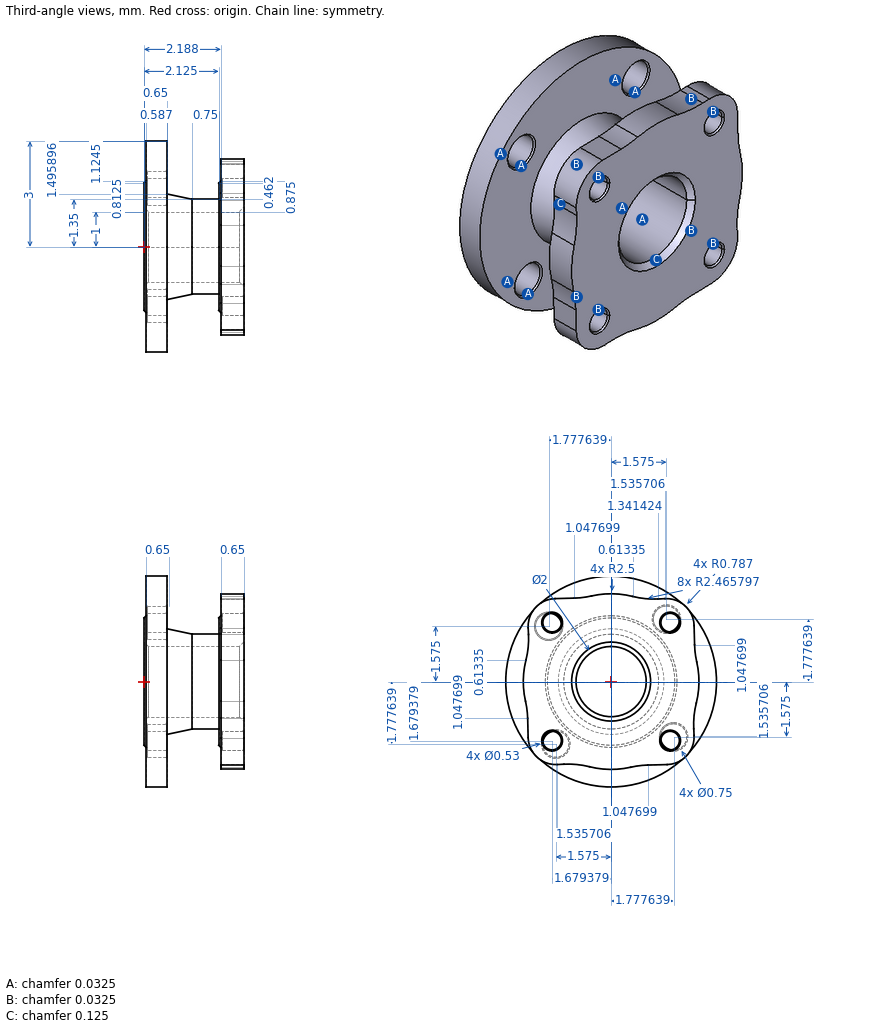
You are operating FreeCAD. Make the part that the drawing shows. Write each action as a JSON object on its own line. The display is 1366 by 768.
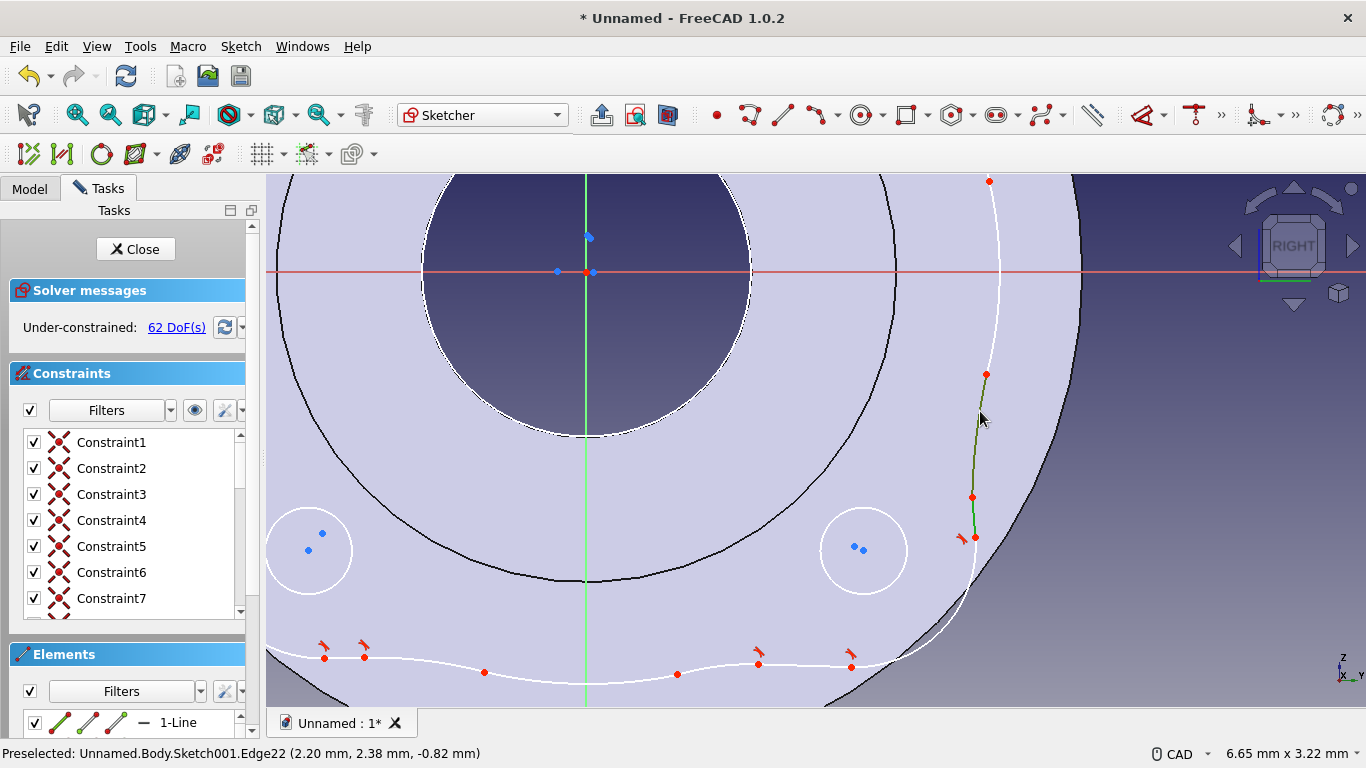
{"action": "key", "text": "t"}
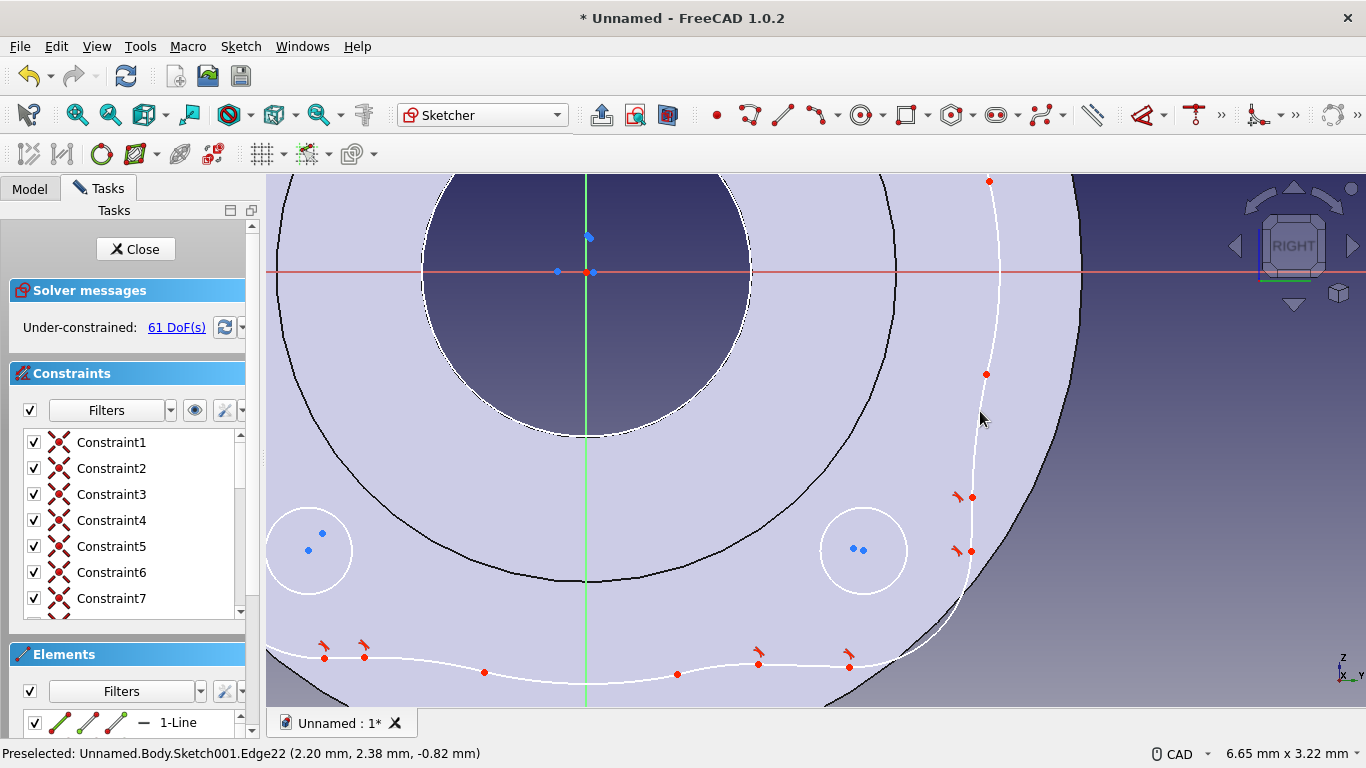
{"action": "scroll", "coordinate": [879, 578], "scroll_direction": "down", "scroll_amount": 4}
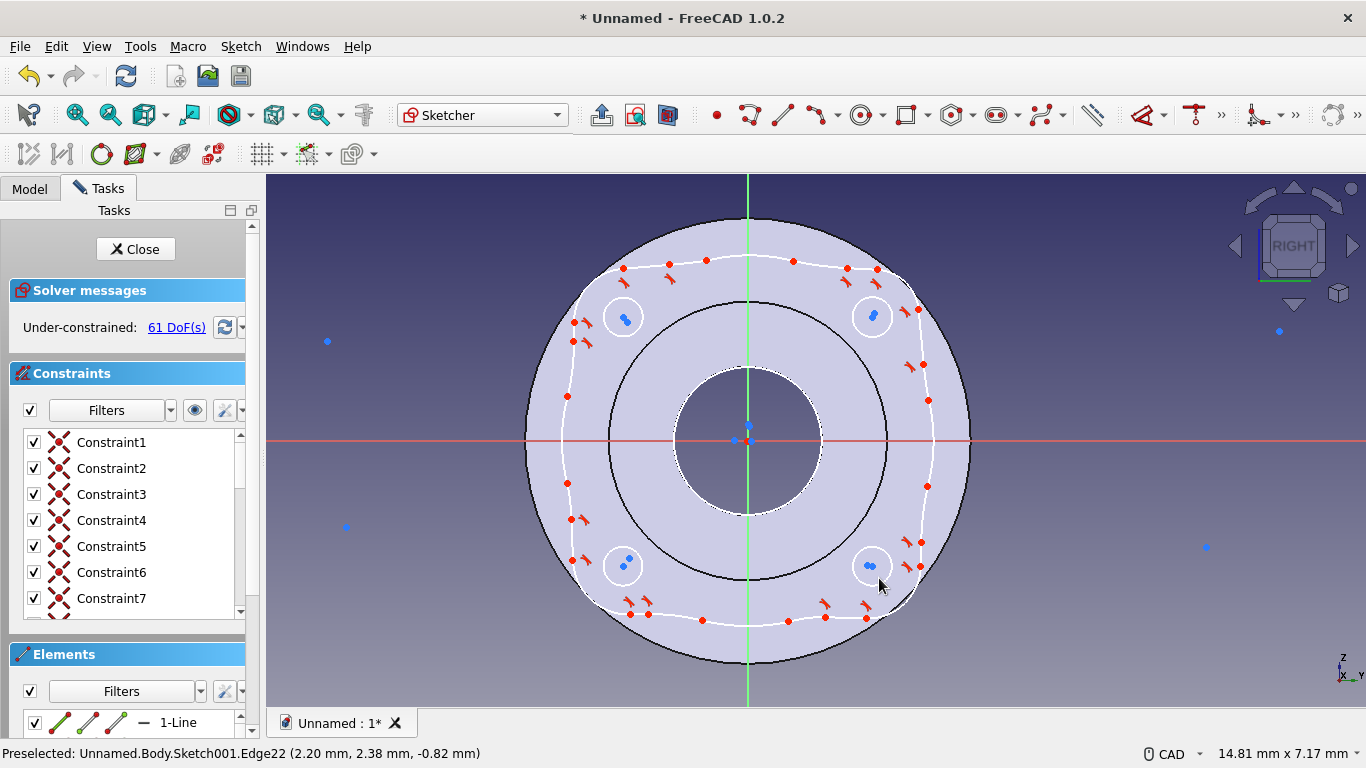
{"action": "left_click", "coordinate": [809, 264]}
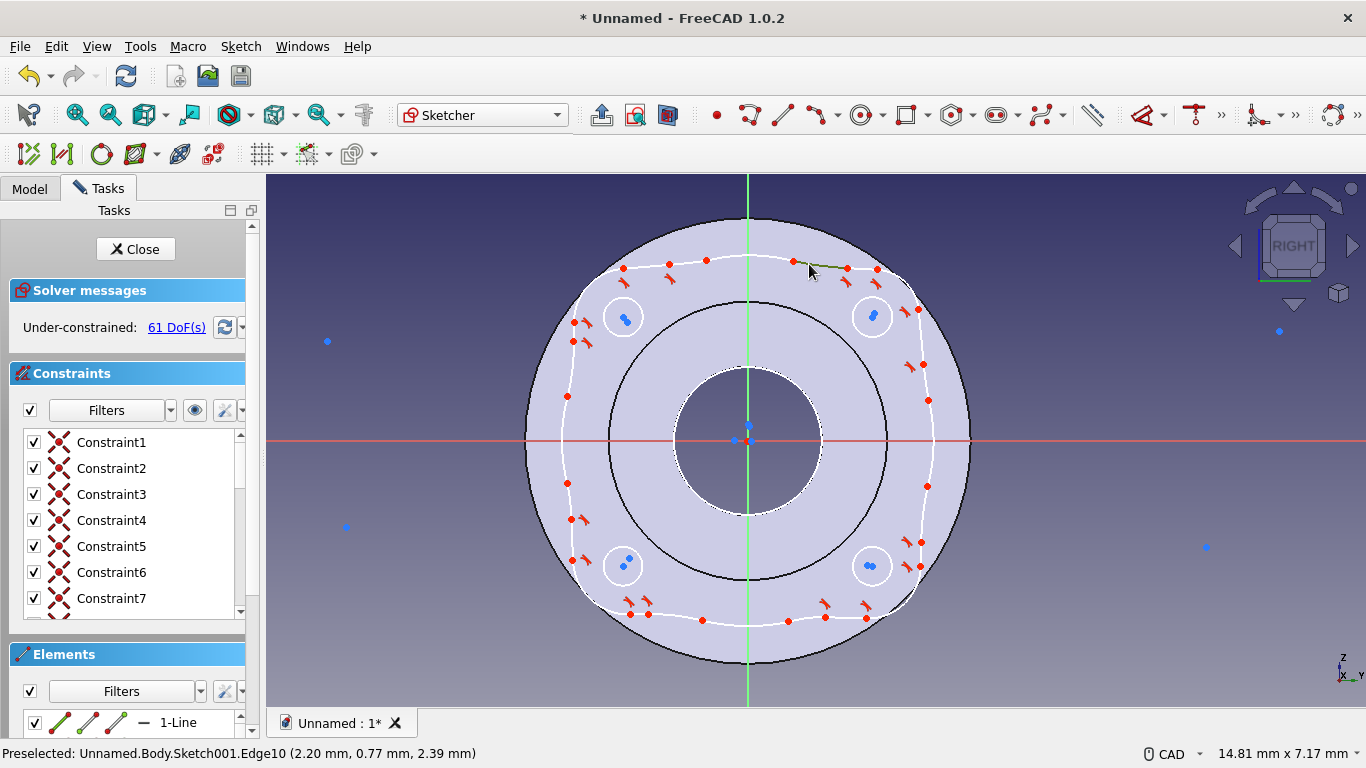
{"action": "left_click", "coordinate": [767, 256]}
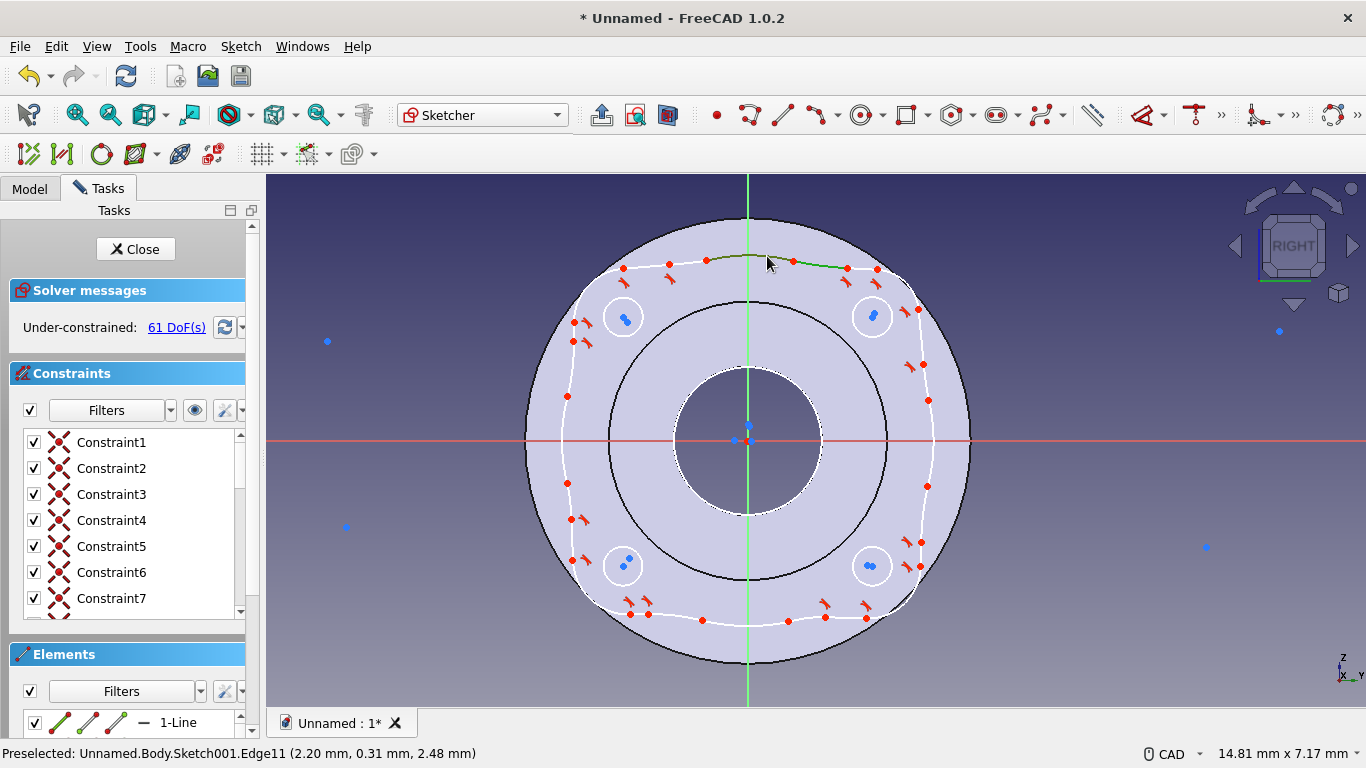
{"action": "key", "text": "t"}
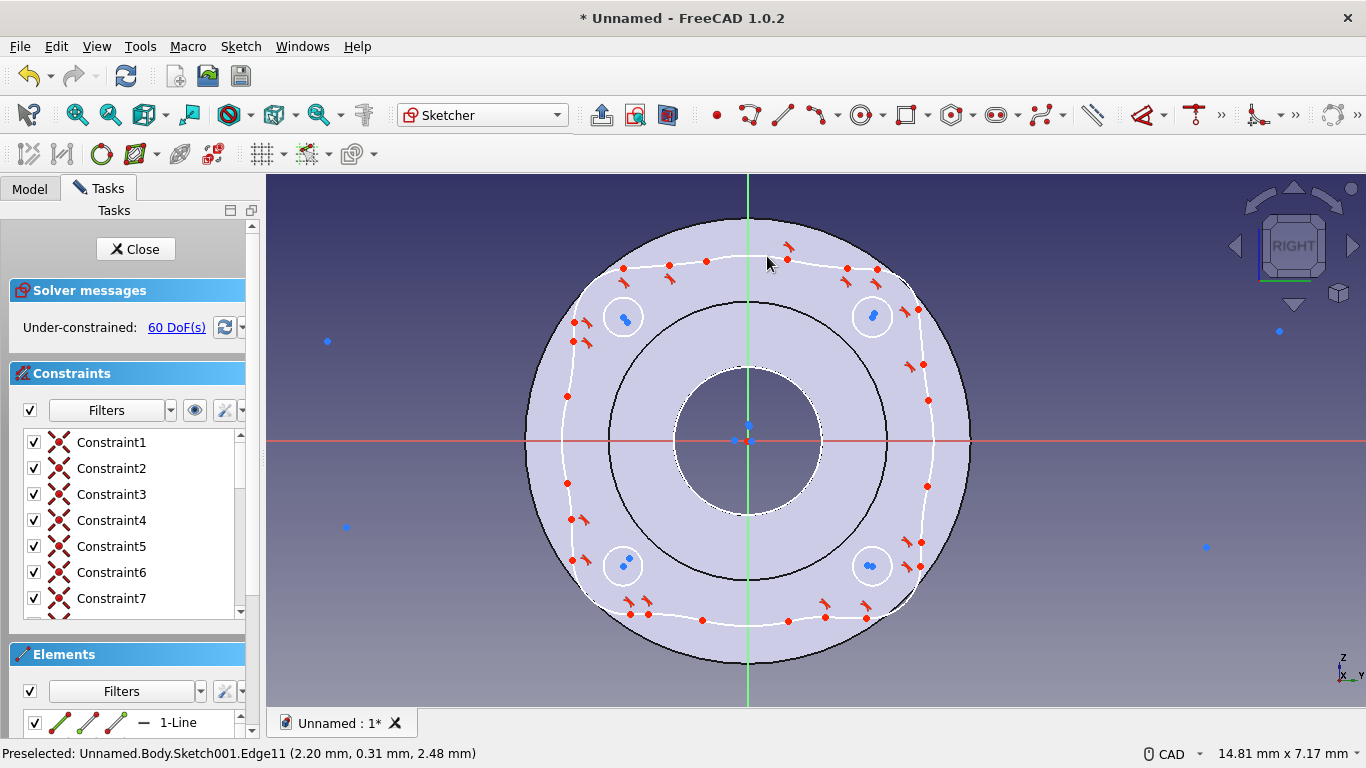
{"action": "left_click", "coordinate": [763, 256]}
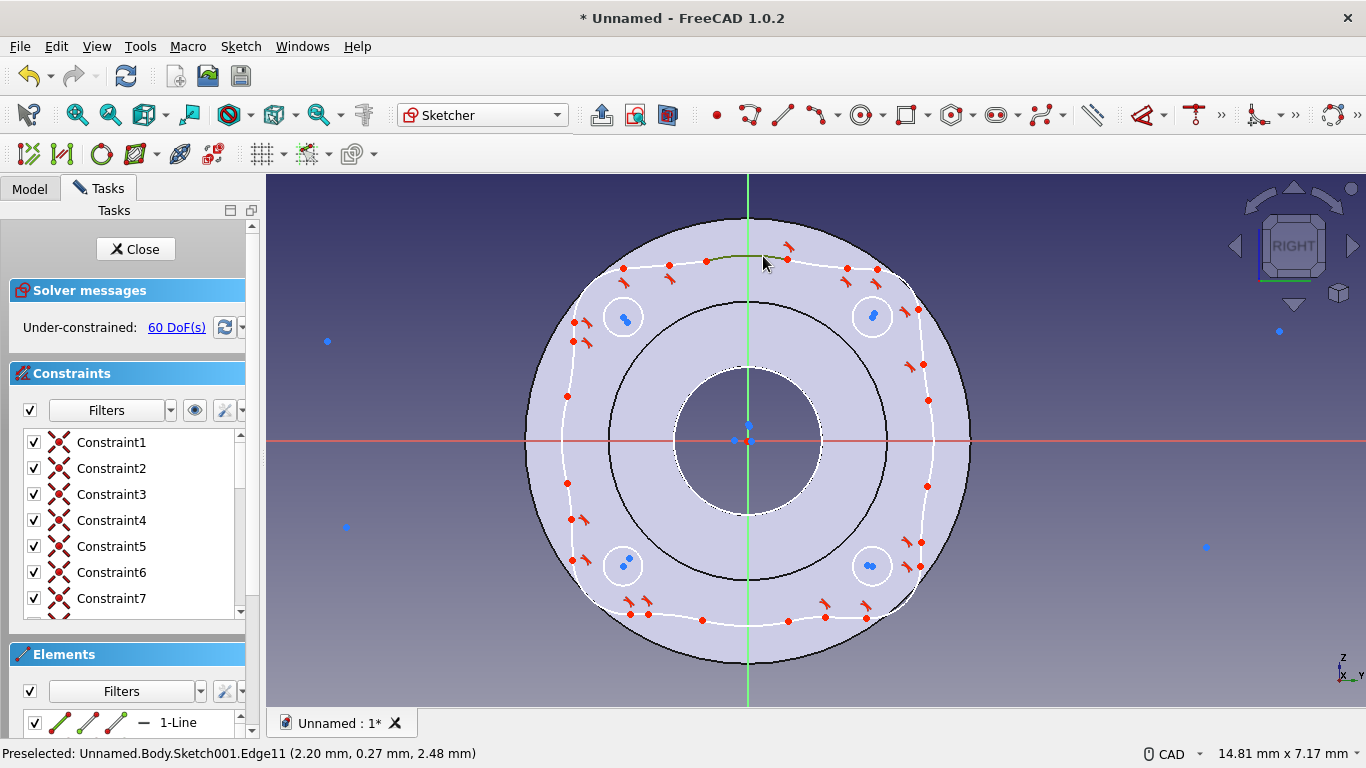
{"action": "scroll", "coordinate": [681, 264], "scroll_direction": "up", "scroll_amount": 2}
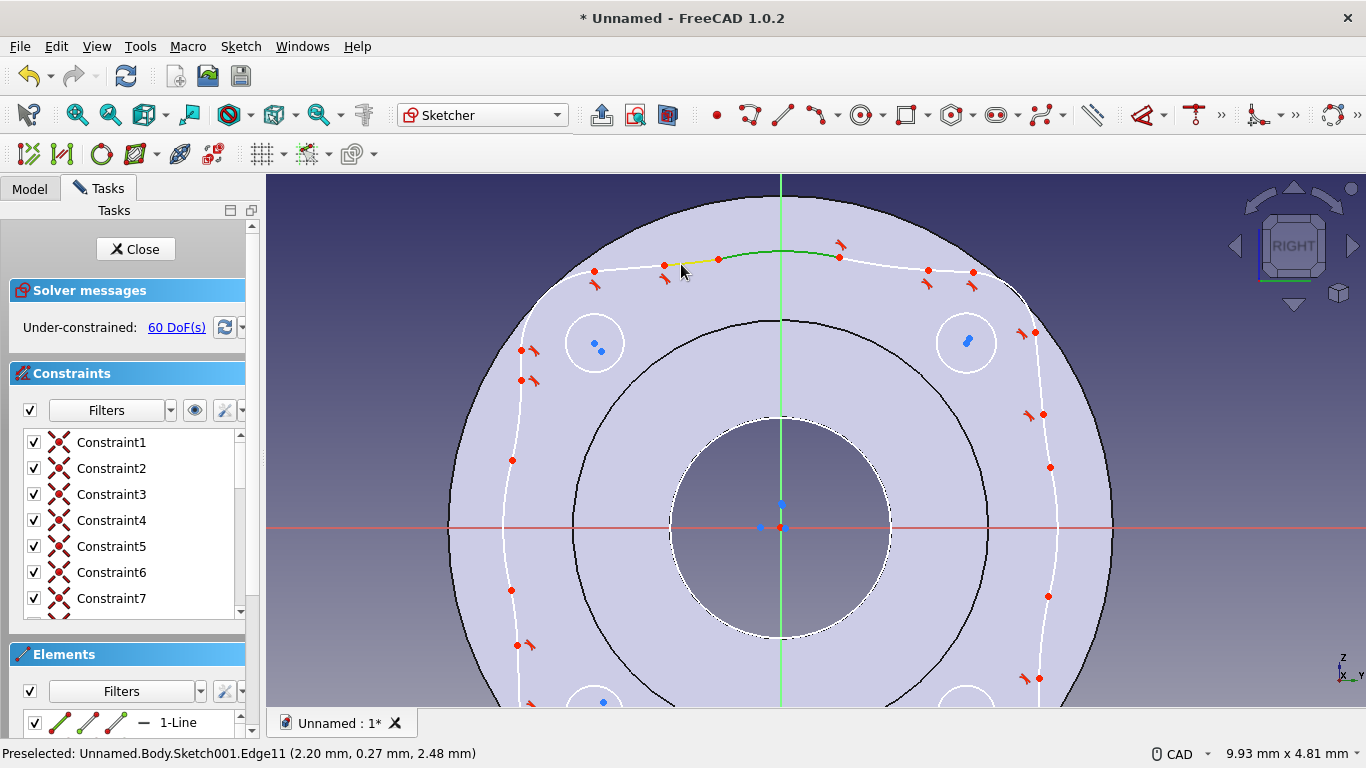
{"action": "left_click", "coordinate": [681, 264]}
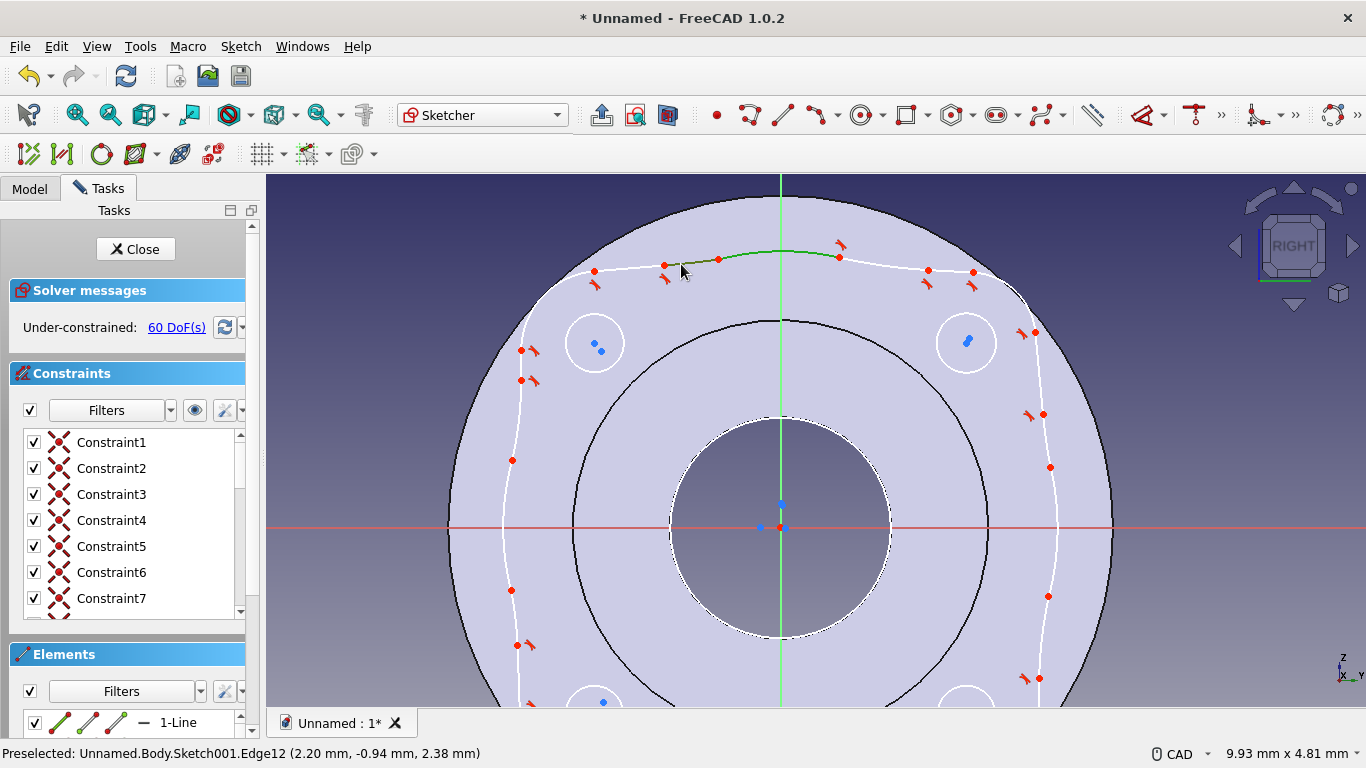
{"action": "key", "text": "t"}